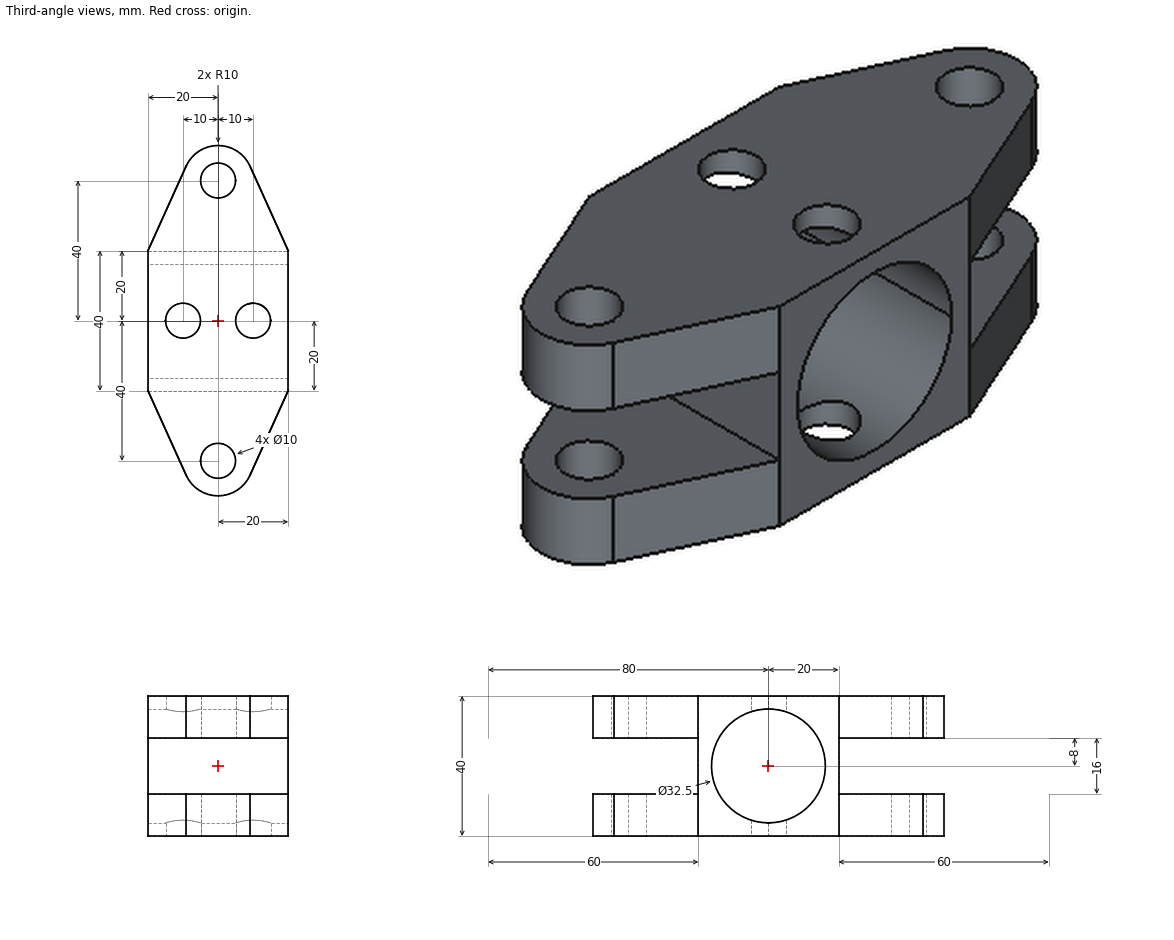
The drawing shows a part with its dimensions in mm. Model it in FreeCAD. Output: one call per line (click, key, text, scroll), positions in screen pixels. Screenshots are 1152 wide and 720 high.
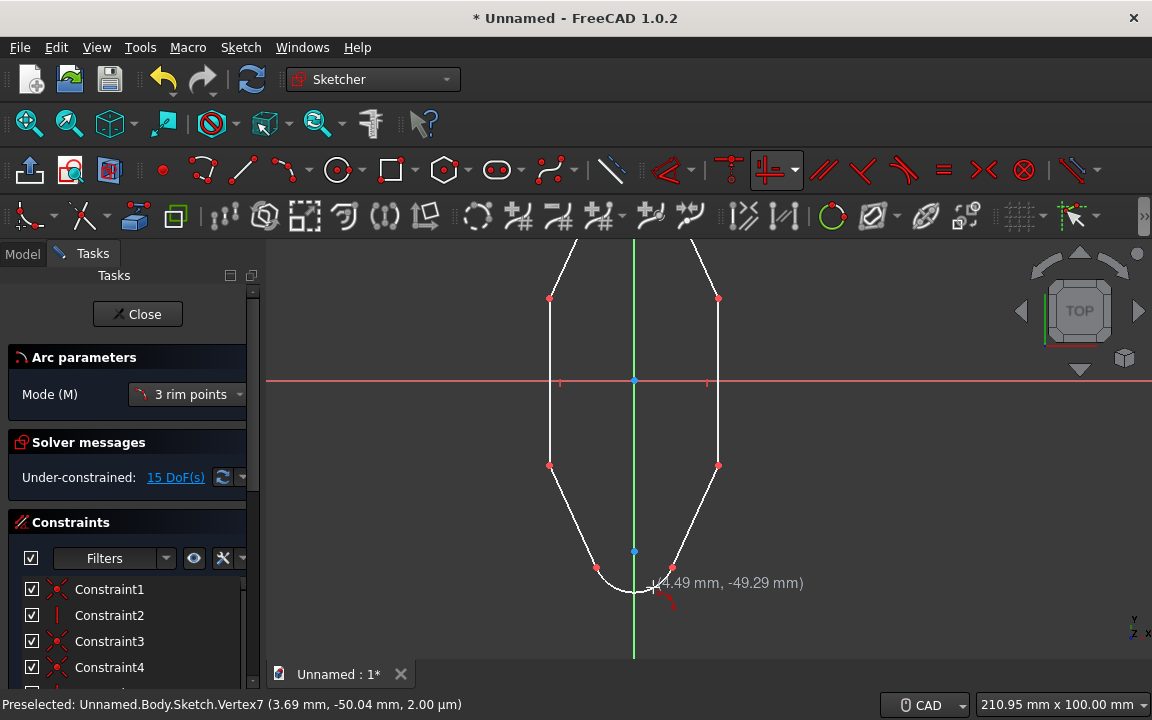
scroll(653, 587, down, 2)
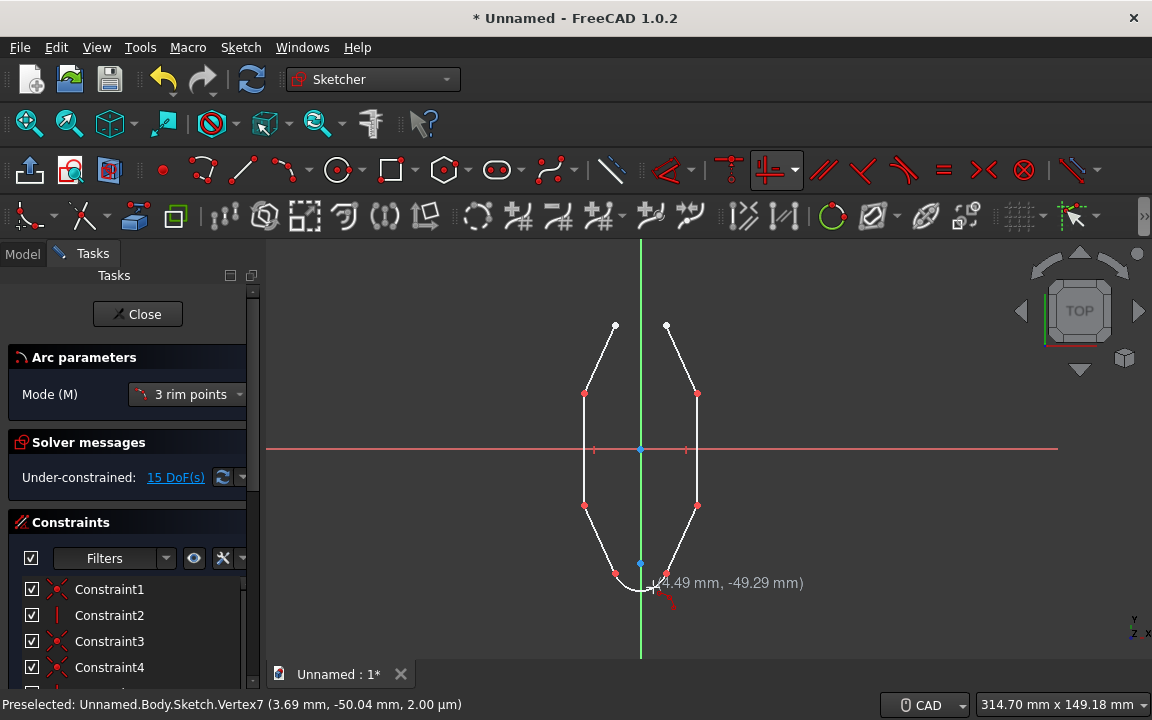
click(666, 326)
click(615, 326)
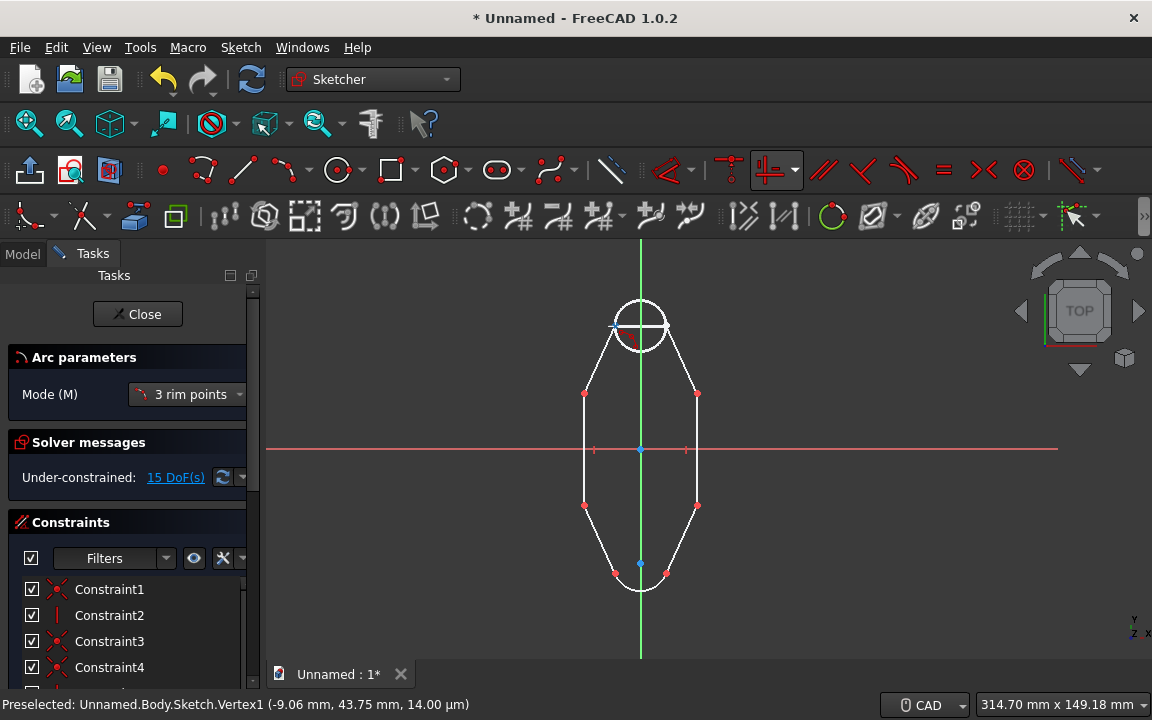
scroll(653, 311, up, 2)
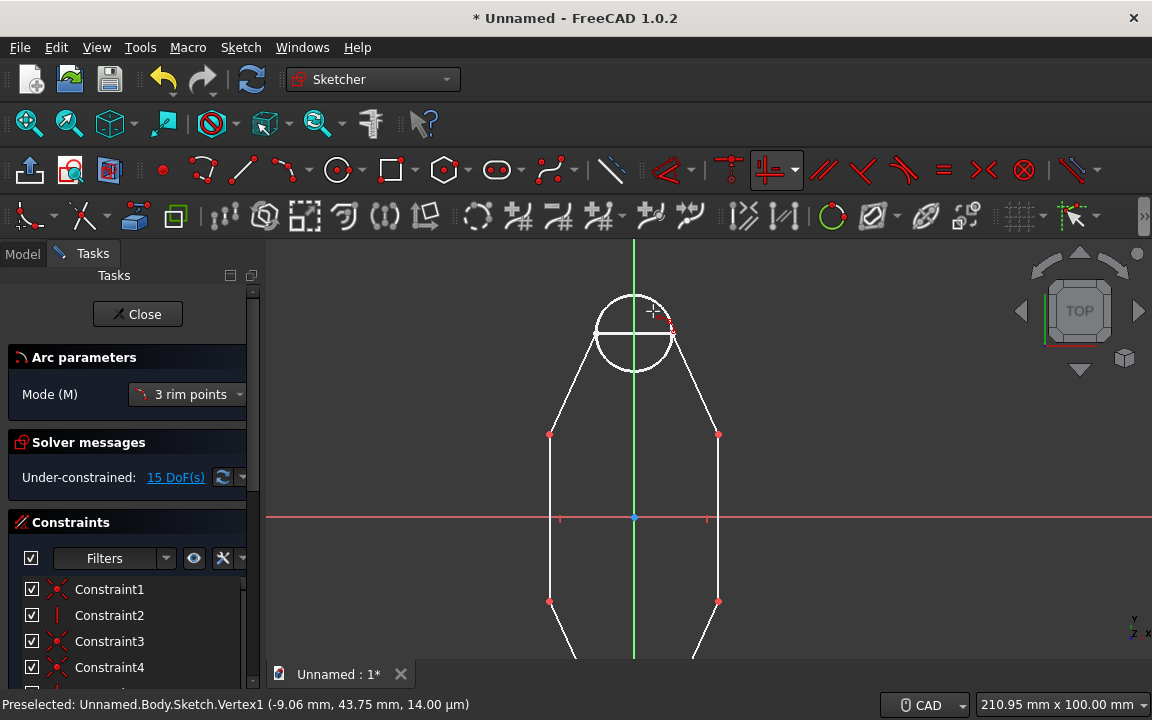
click(653, 311)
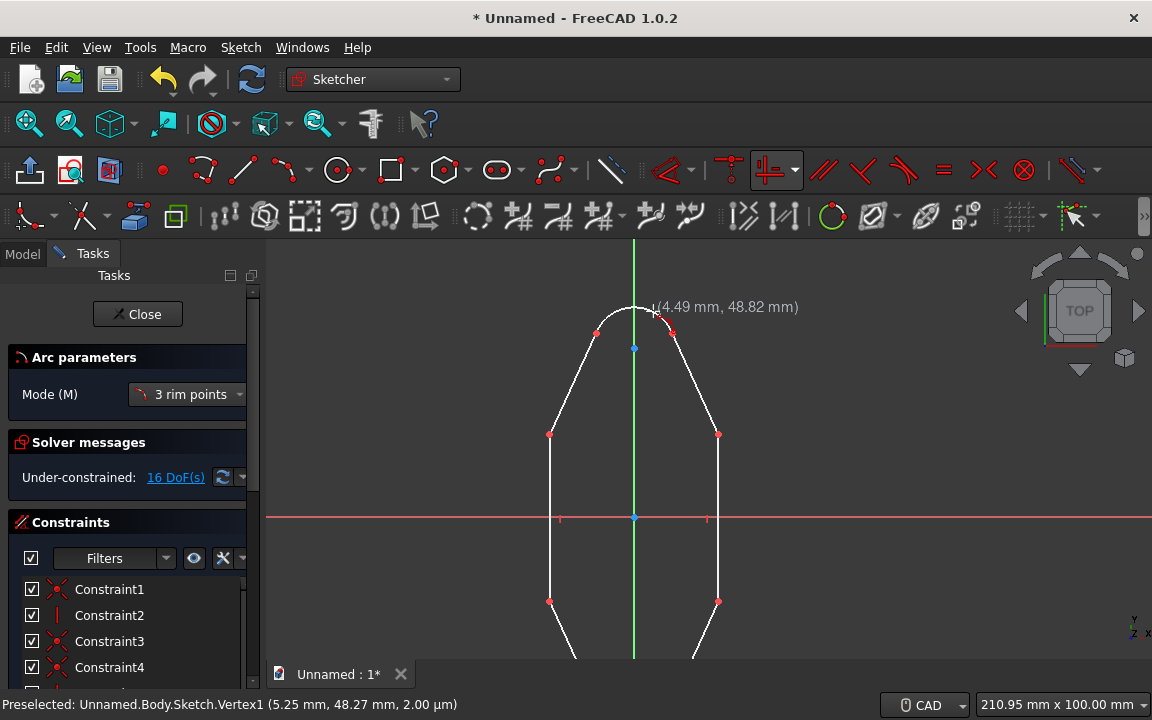
click(338, 170)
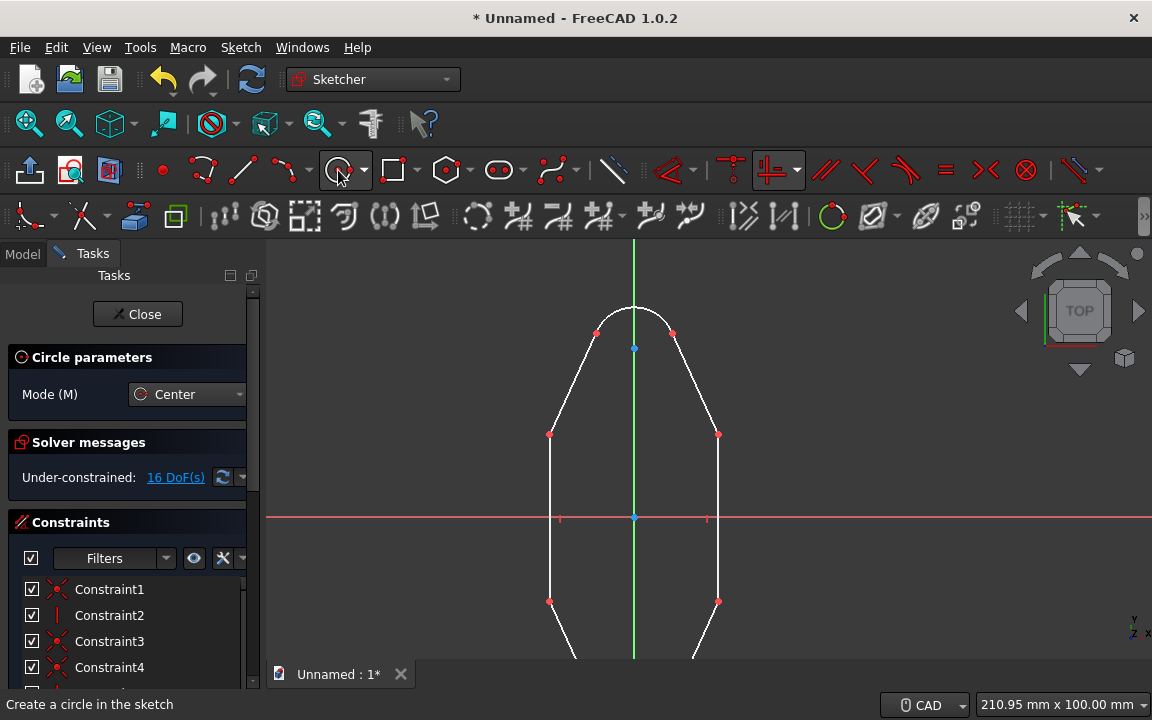
scroll(653, 311, down, 2)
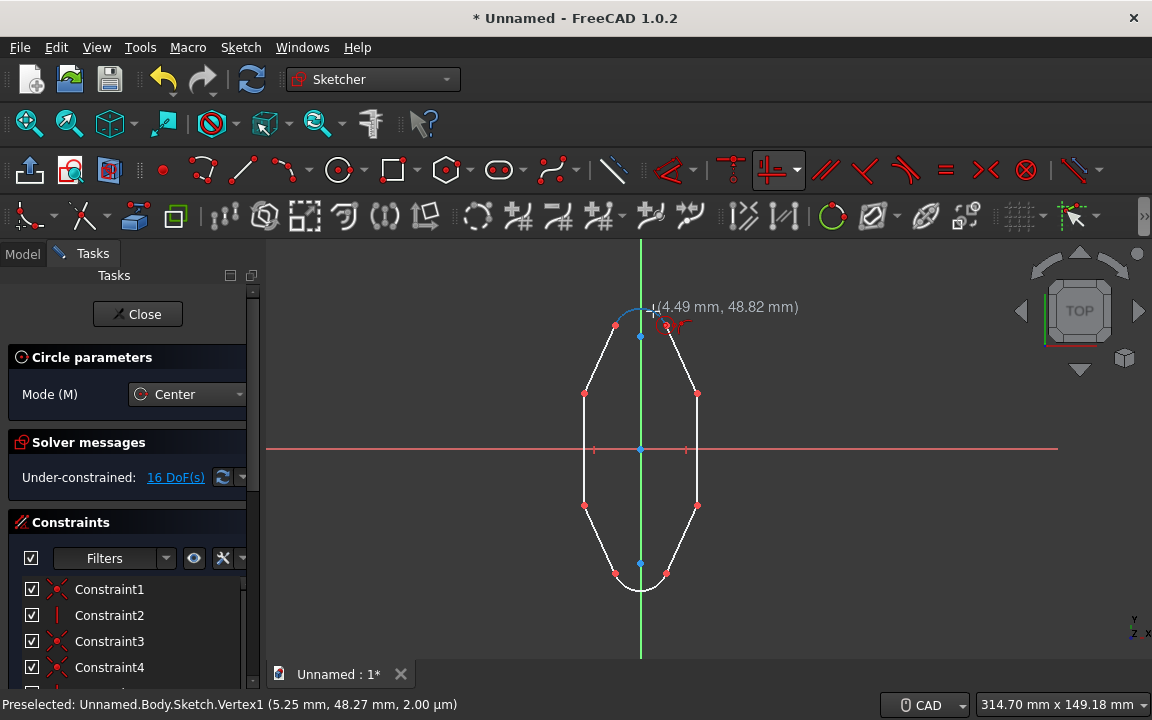
scroll(641, 562, up, 3)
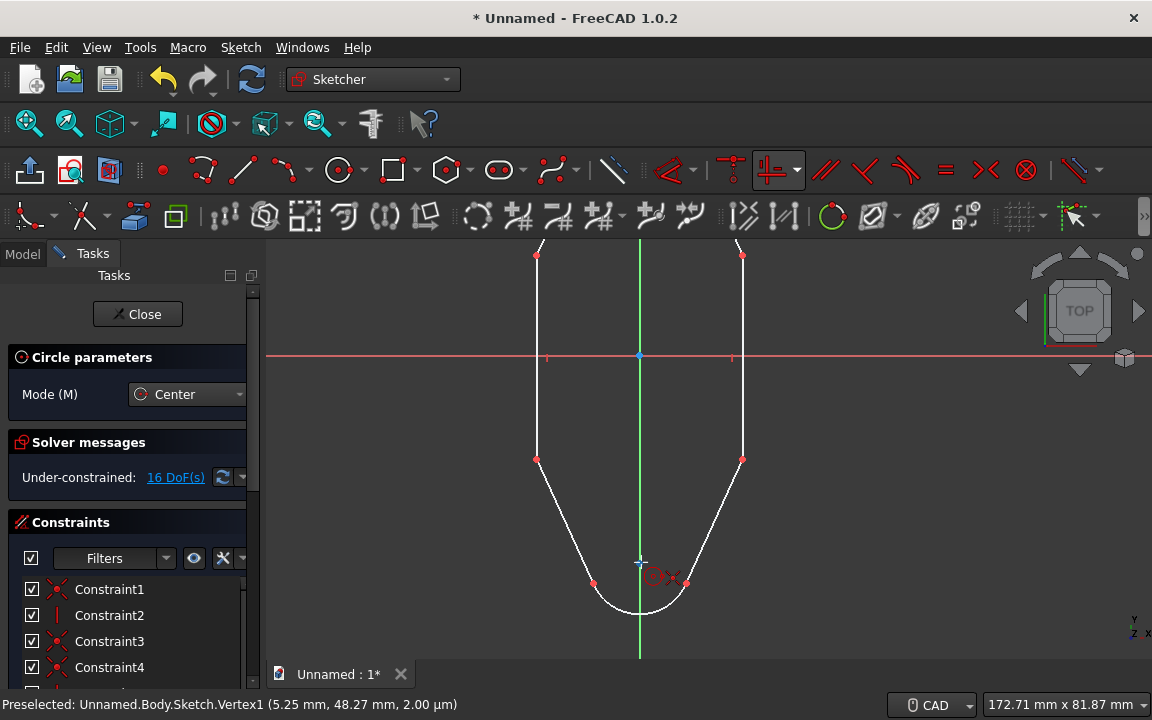
click(640, 561)
move(658, 543)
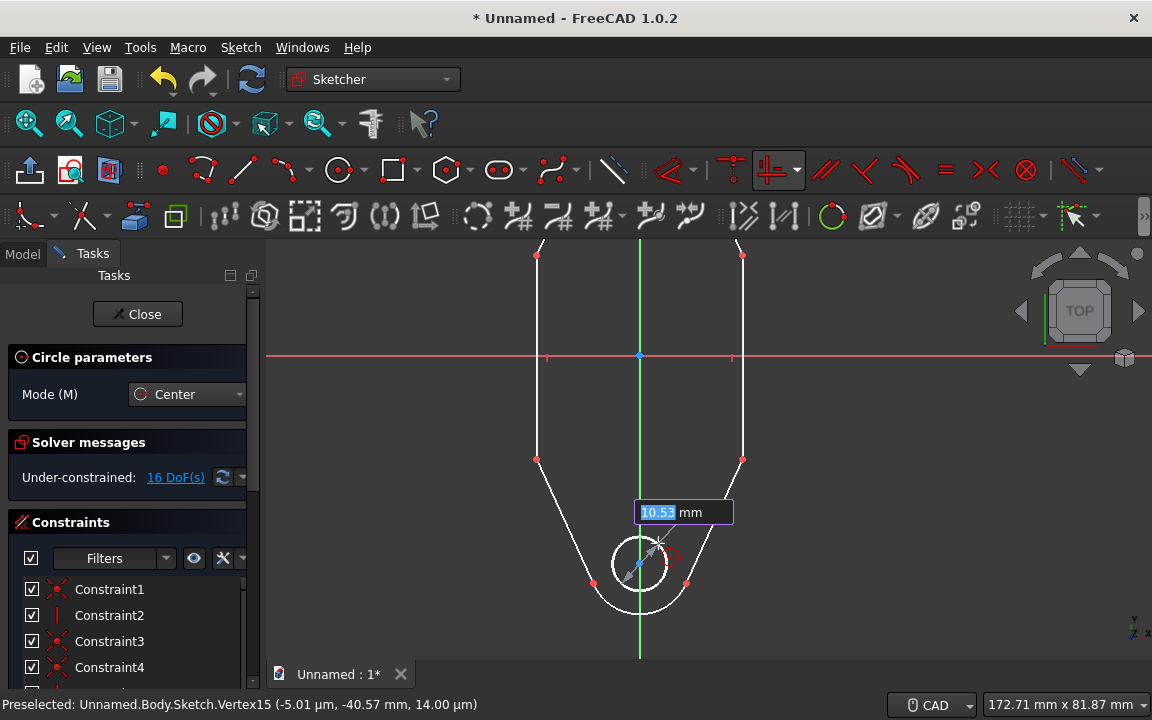
text(10)
key(Return)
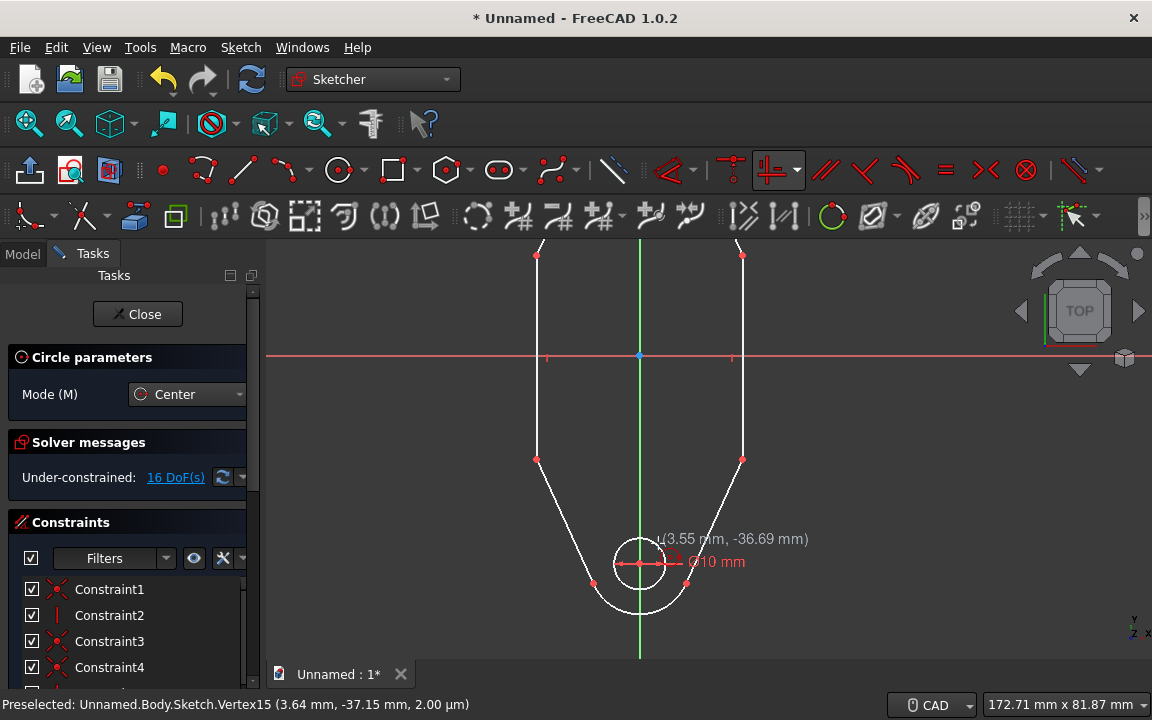
click(588, 356)
move(607, 338)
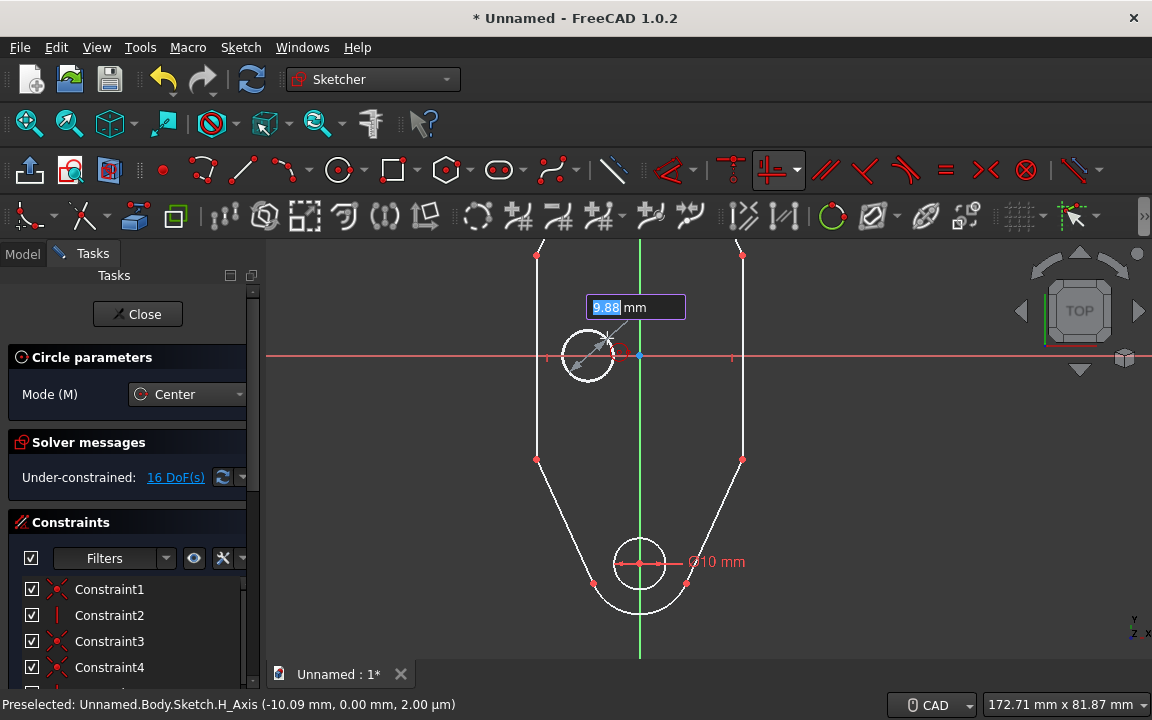
text(10)
key(Return)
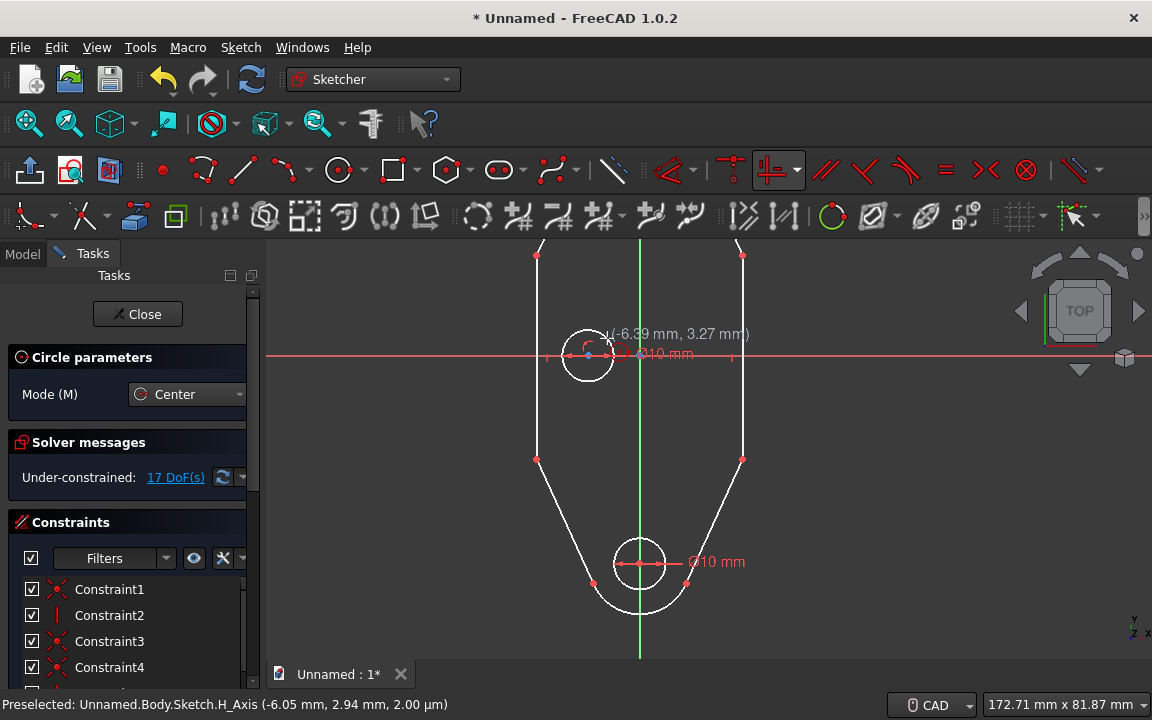
click(691, 356)
move(709, 338)